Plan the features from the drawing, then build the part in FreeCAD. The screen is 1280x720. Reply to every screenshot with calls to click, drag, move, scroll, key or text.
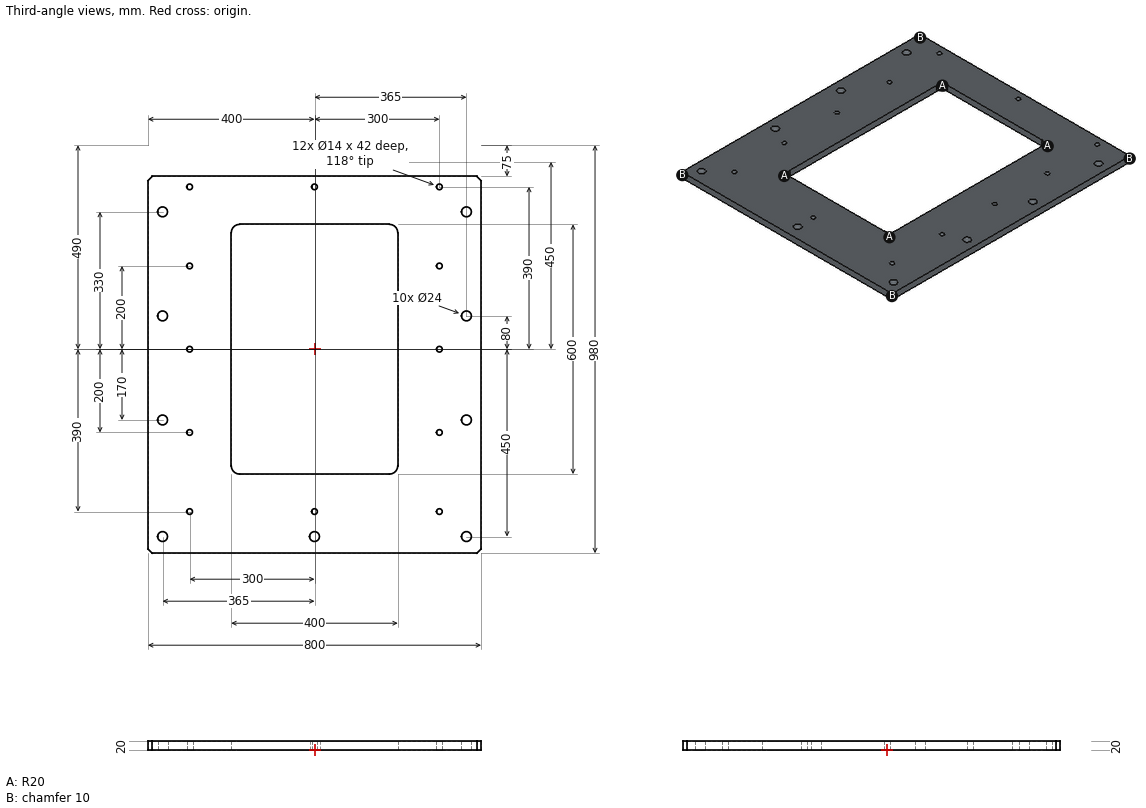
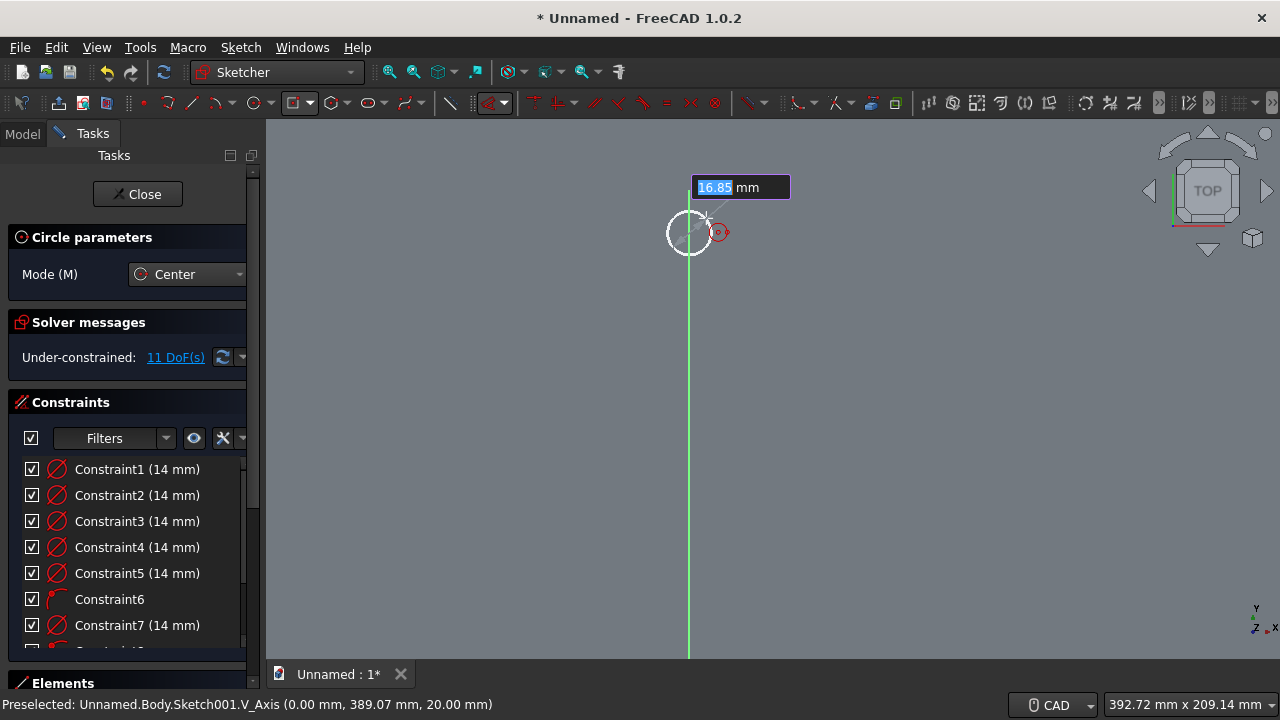
text(14)
key(Return)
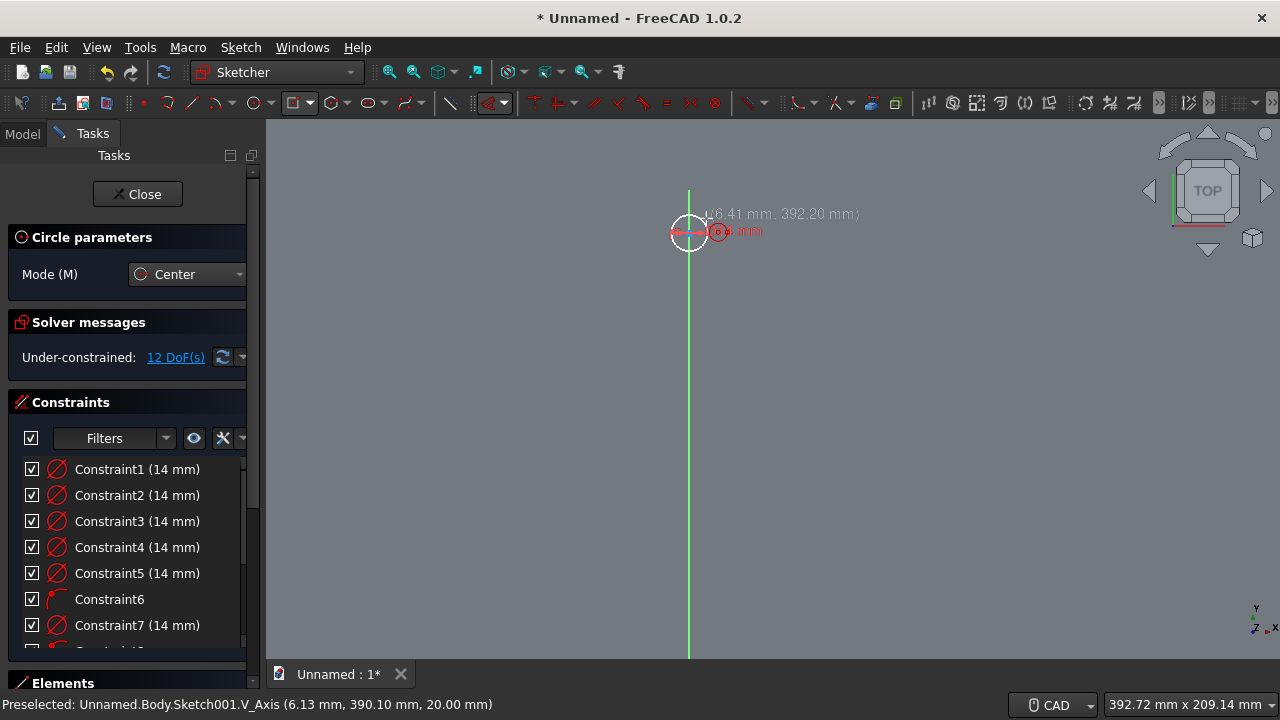
scroll(707, 222, down, 9)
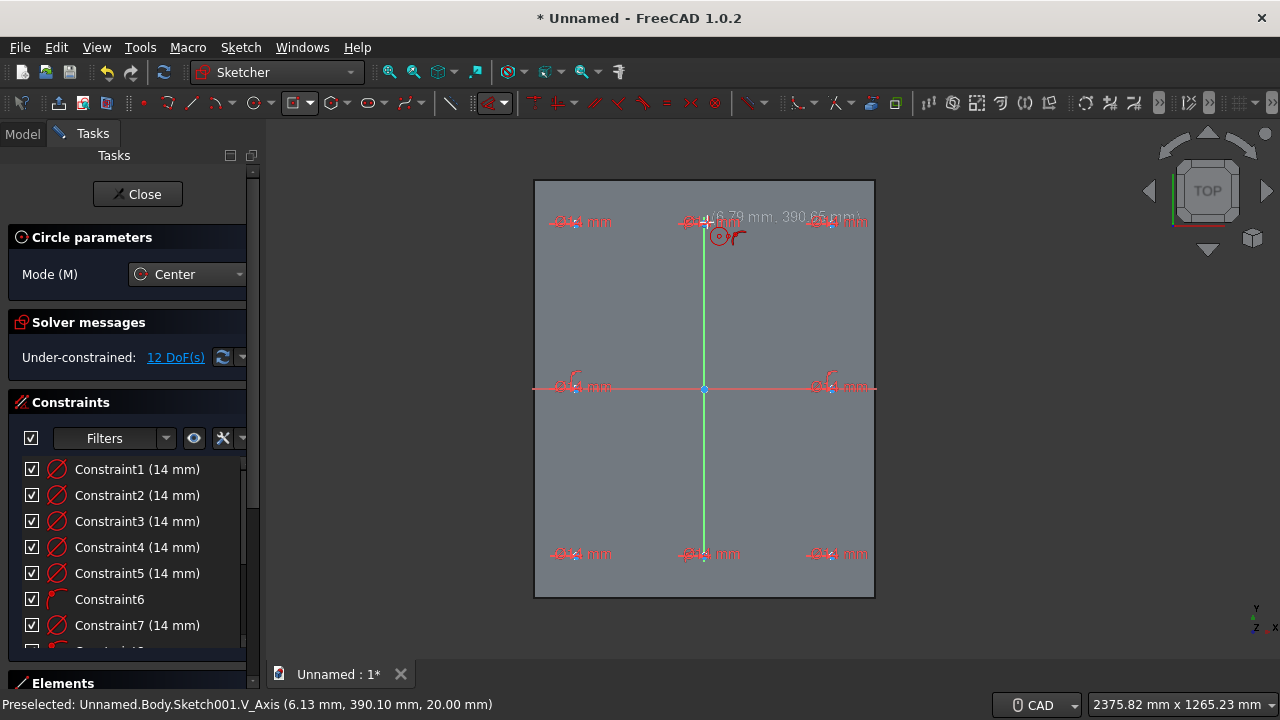
scroll(576, 304, up, 11)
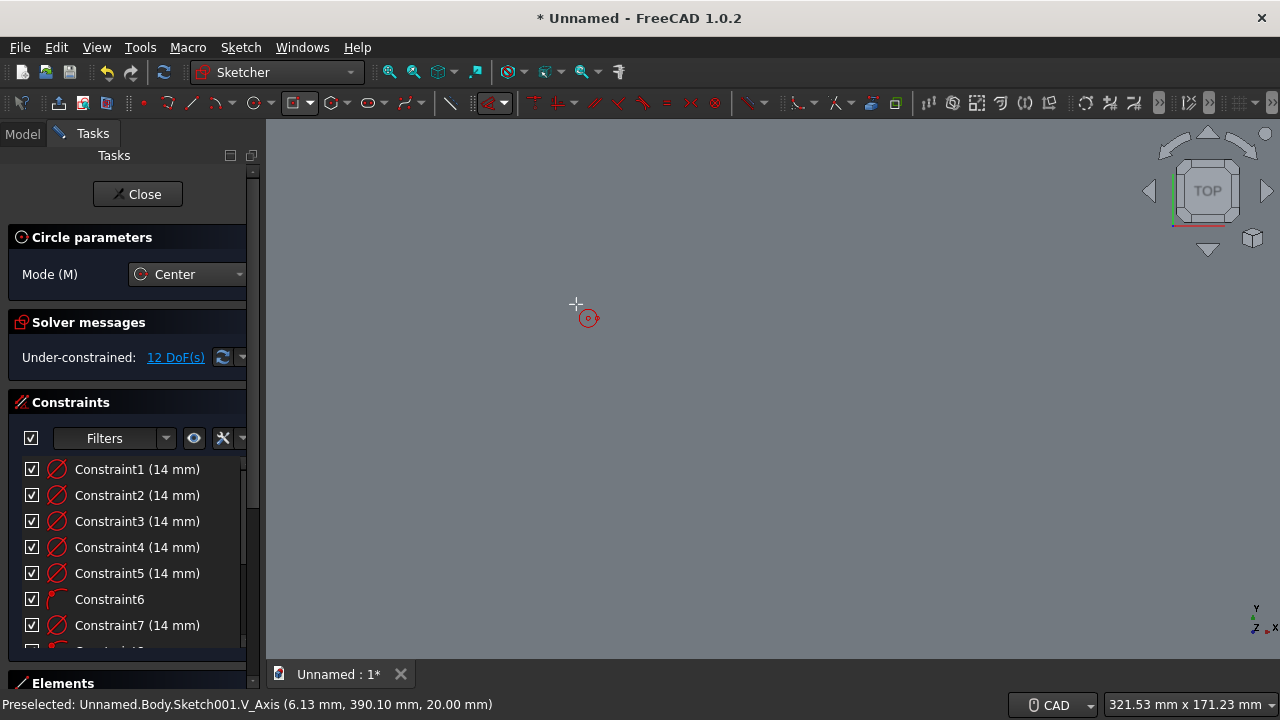
scroll(576, 304, down, 11)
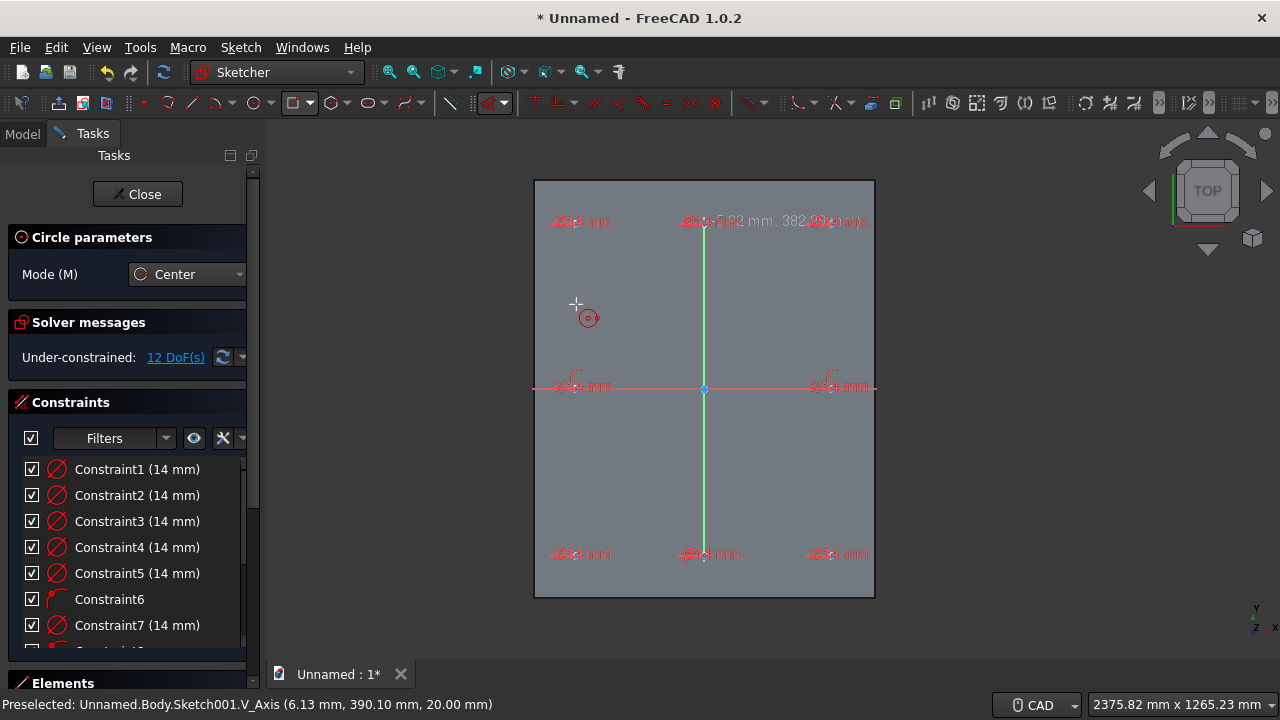
click(576, 304)
move(579, 302)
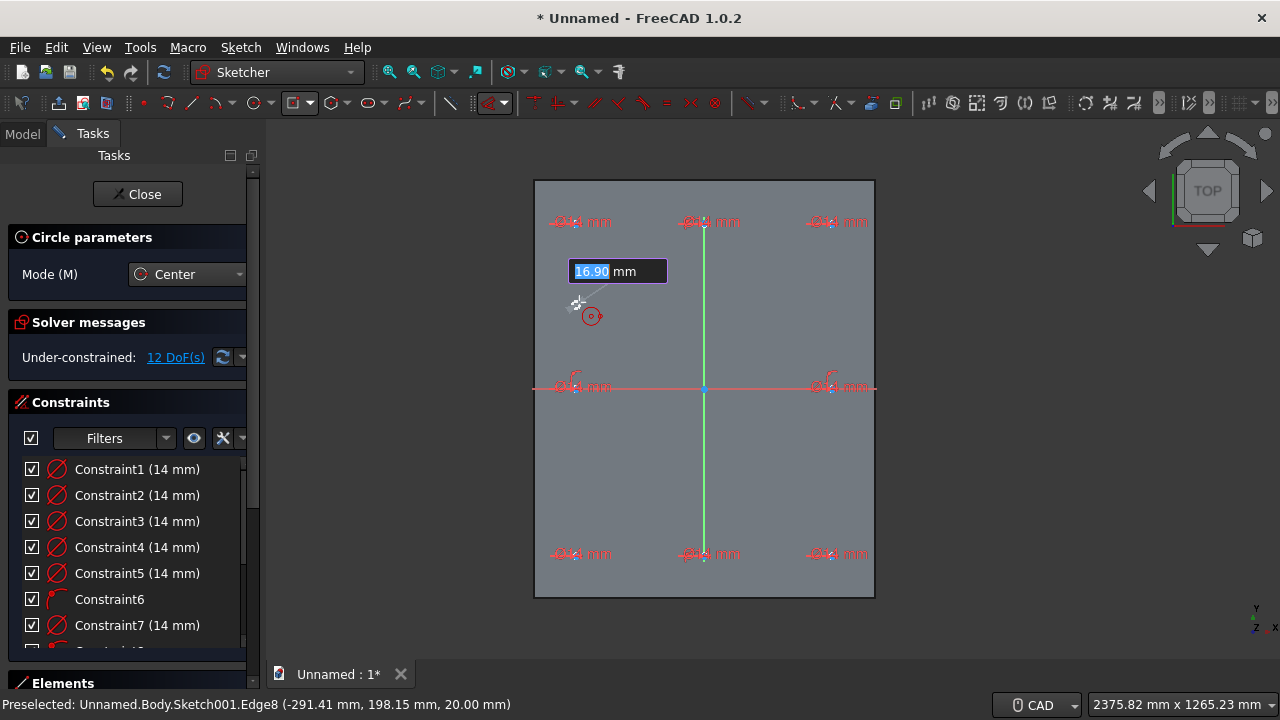
text(14)
key(Return)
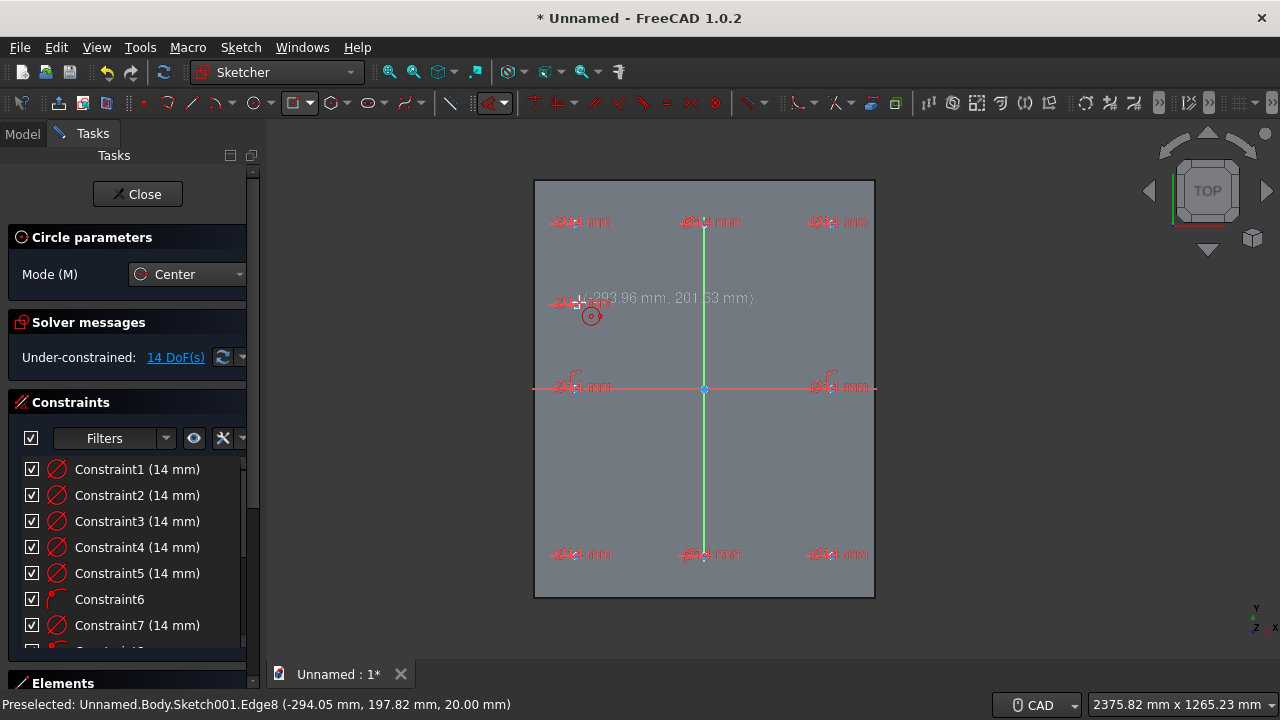
scroll(833, 304, up, 11)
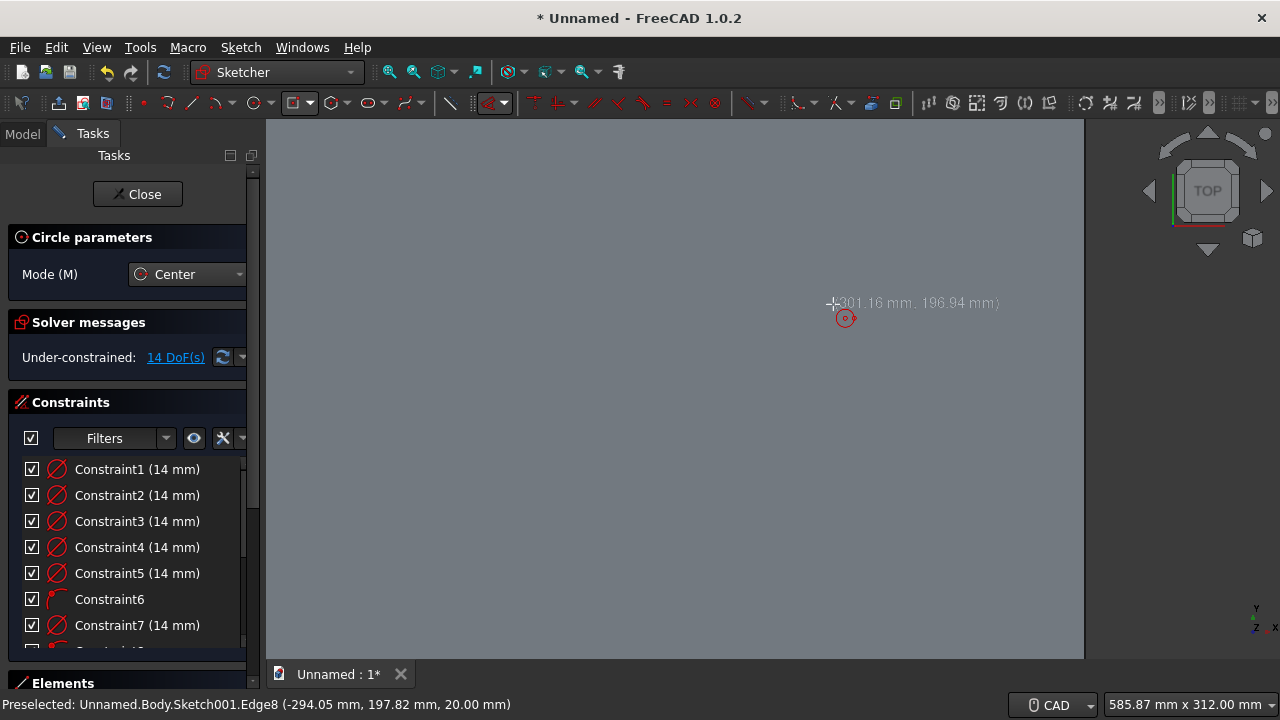
scroll(834, 304, down, 11)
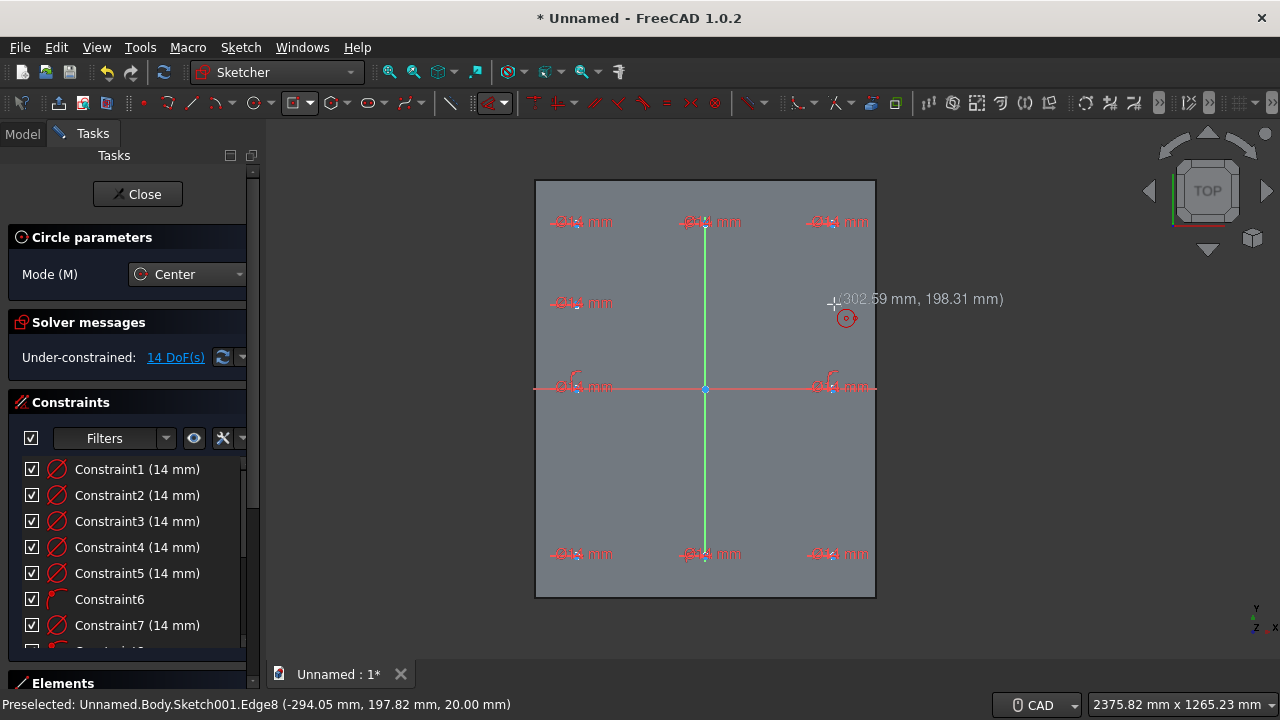
click(833, 304)
move(836, 302)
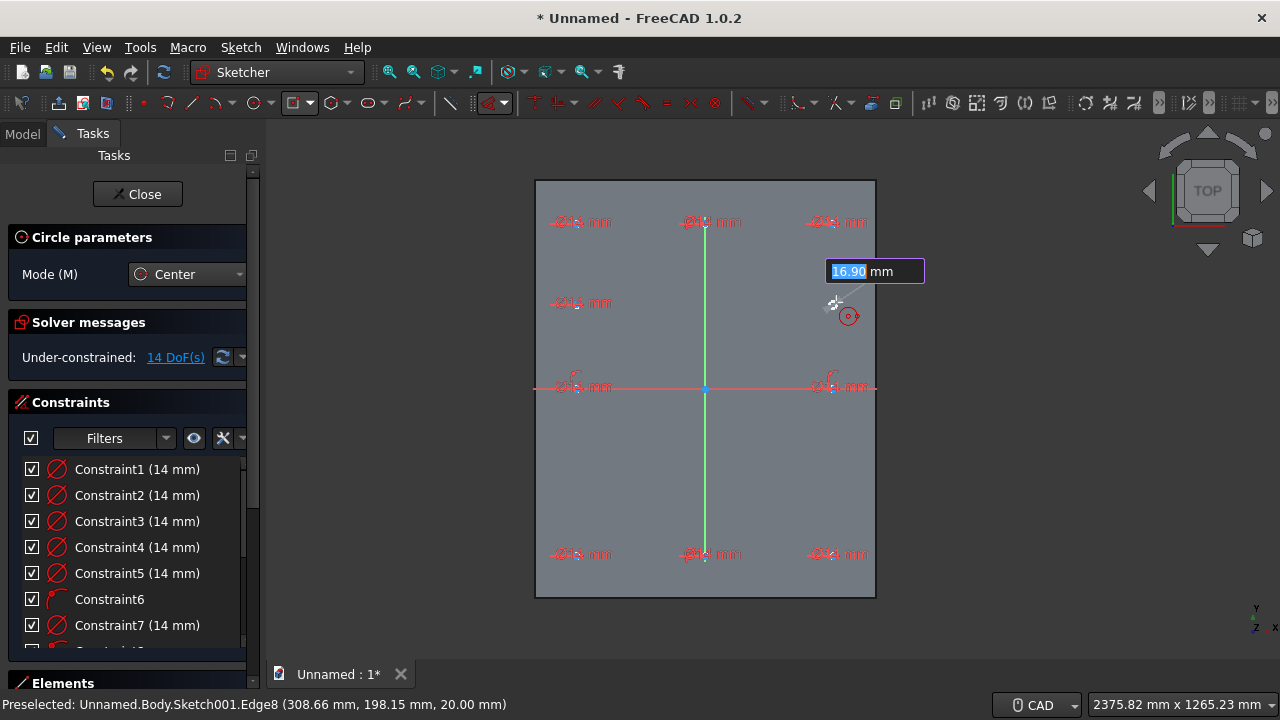
text(14)
key(Return)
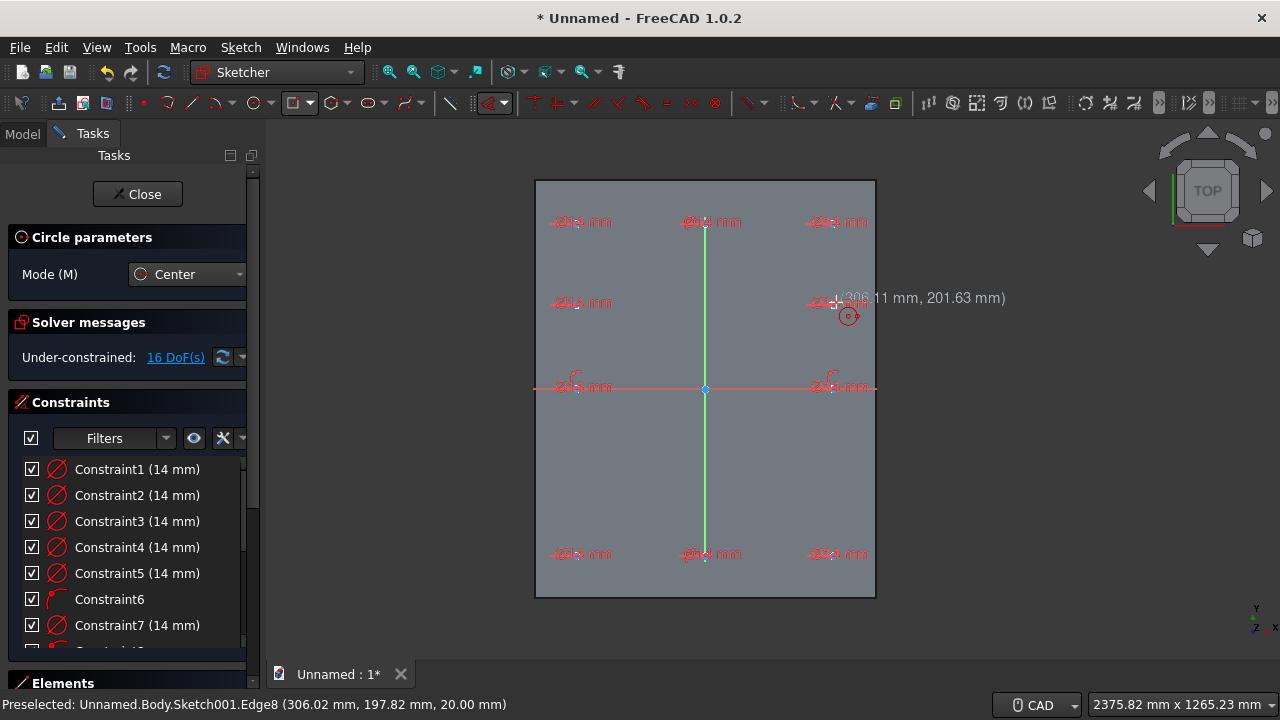
scroll(577, 474, up, 11)